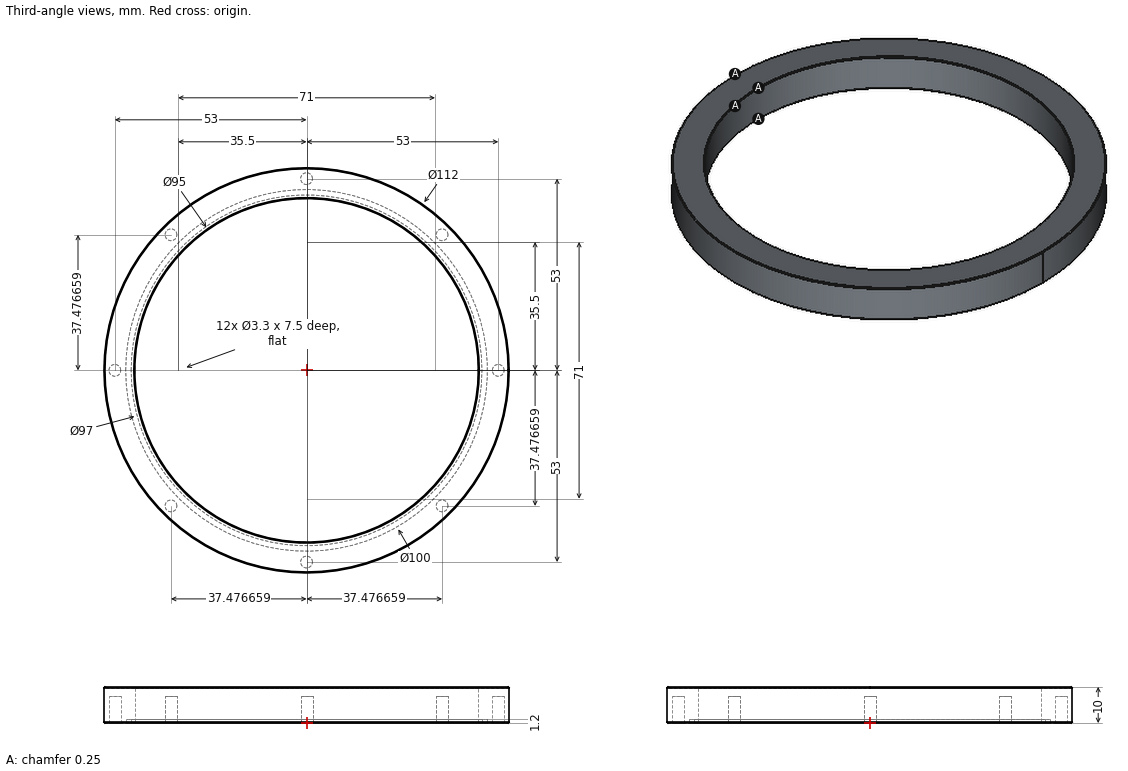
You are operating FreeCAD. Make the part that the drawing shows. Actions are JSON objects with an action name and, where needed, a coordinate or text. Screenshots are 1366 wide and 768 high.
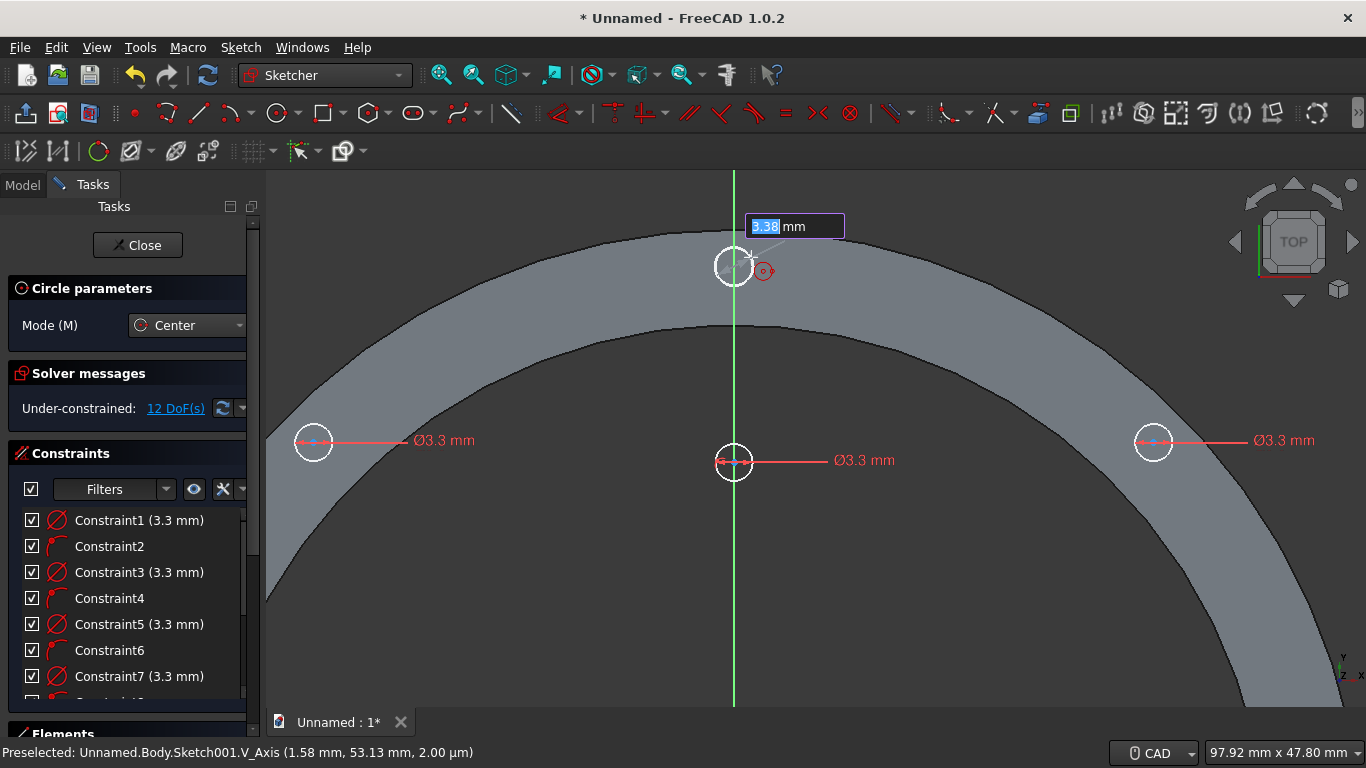
{"action": "type", "text": "3.3"}
{"action": "key", "text": "Return"}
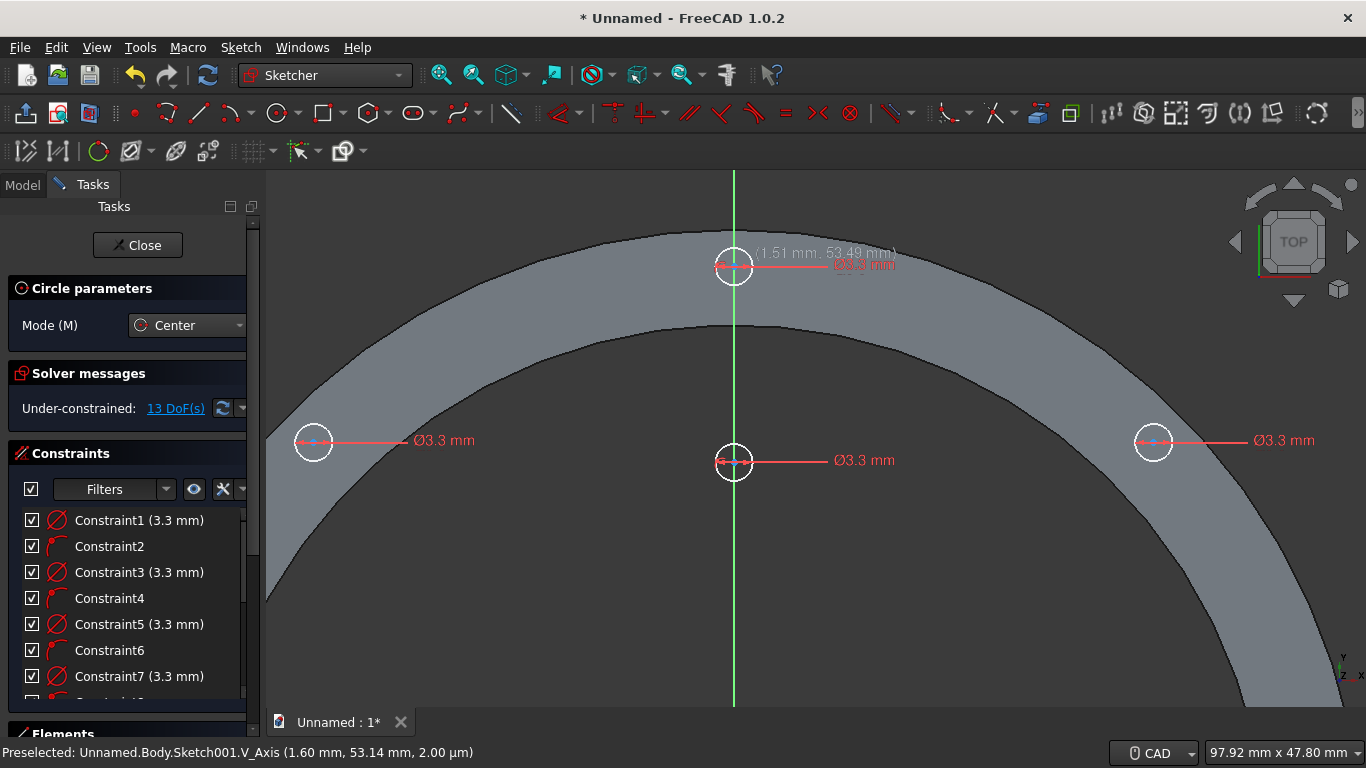
{"action": "scroll", "coordinate": [753, 257], "scroll_direction": "down", "scroll_amount": 6}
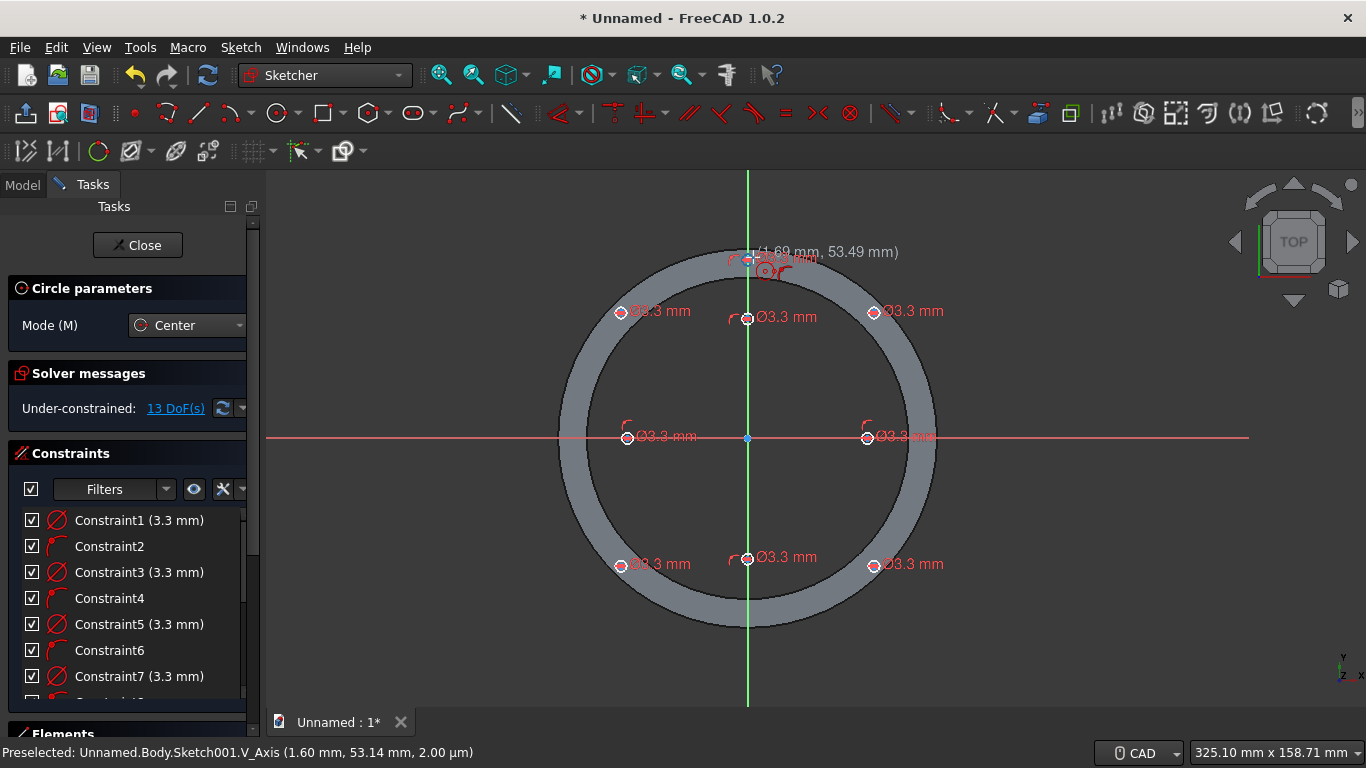
{"action": "scroll", "coordinate": [568, 438], "scroll_direction": "up", "scroll_amount": 8}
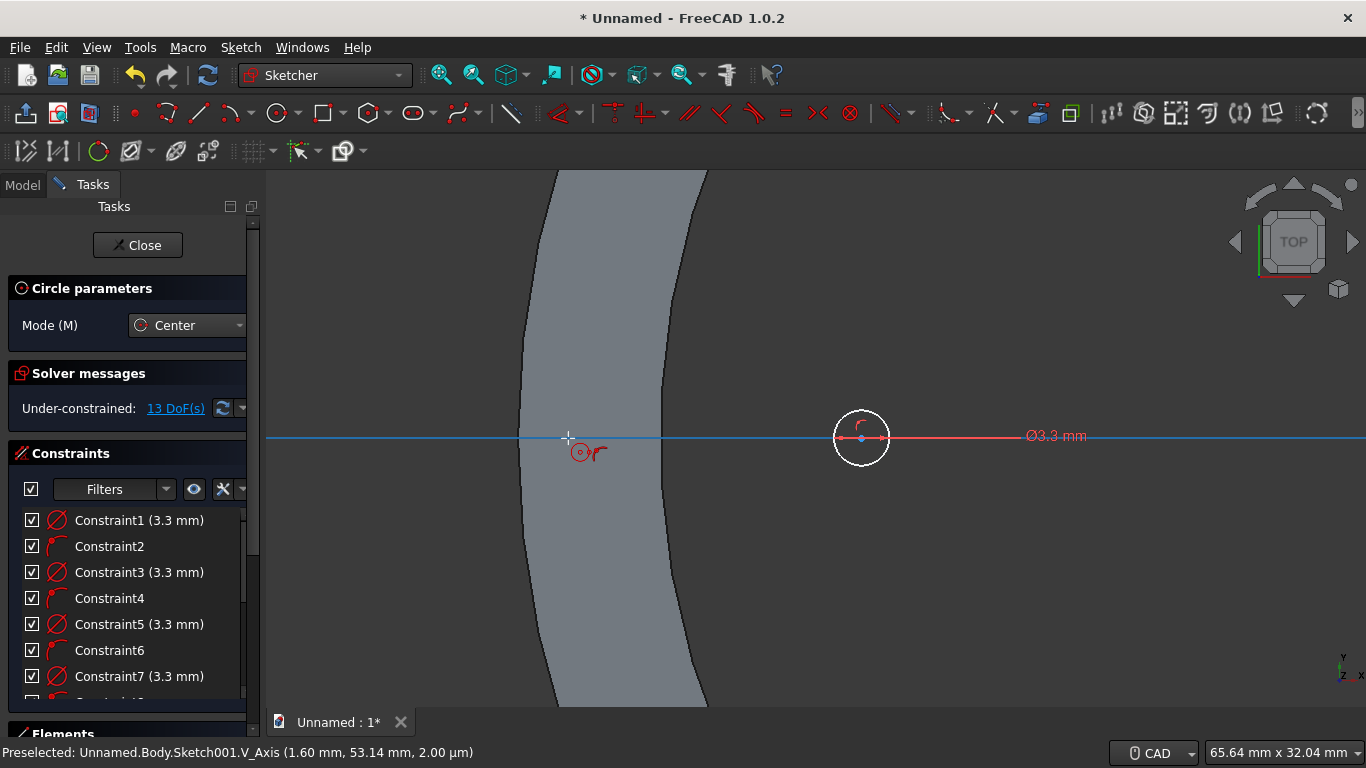
{"action": "scroll", "coordinate": [568, 439], "scroll_direction": "down", "scroll_amount": 8}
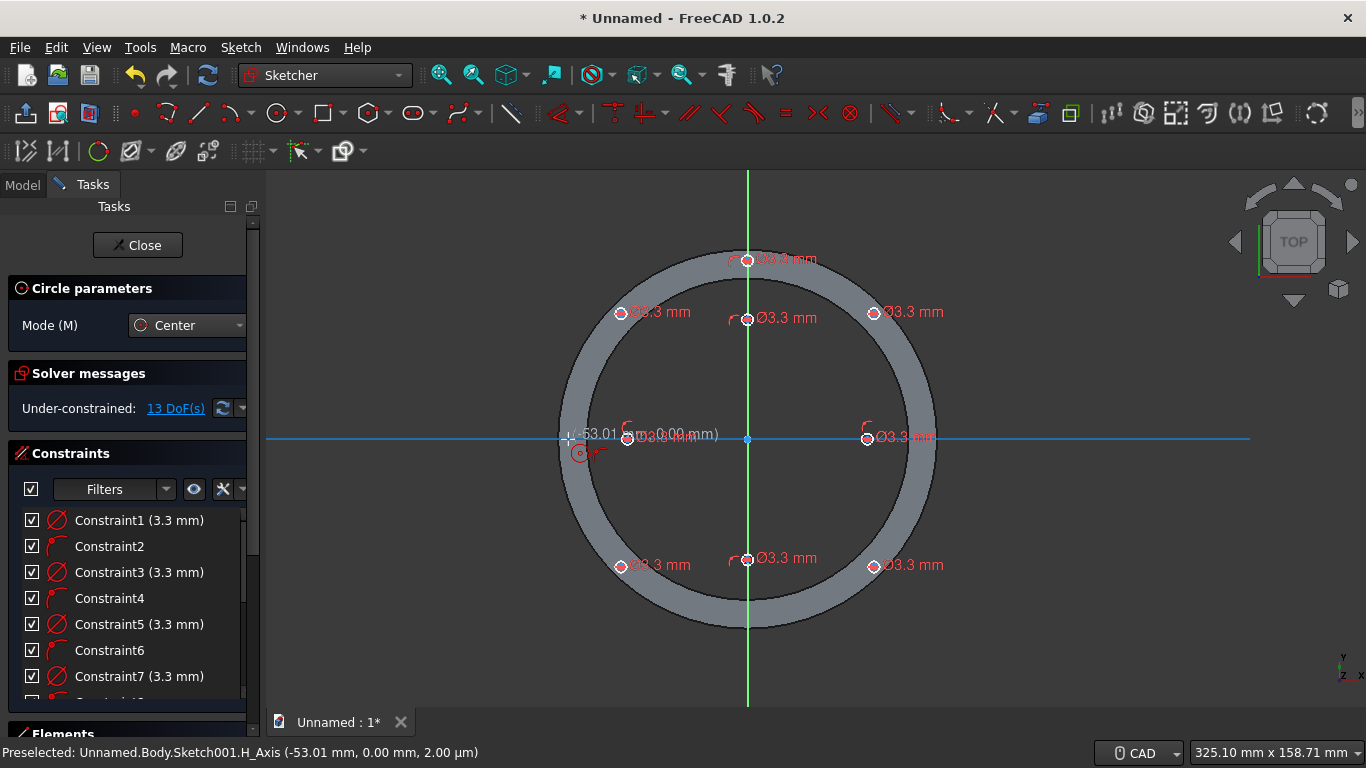
{"action": "left_click", "coordinate": [568, 439]}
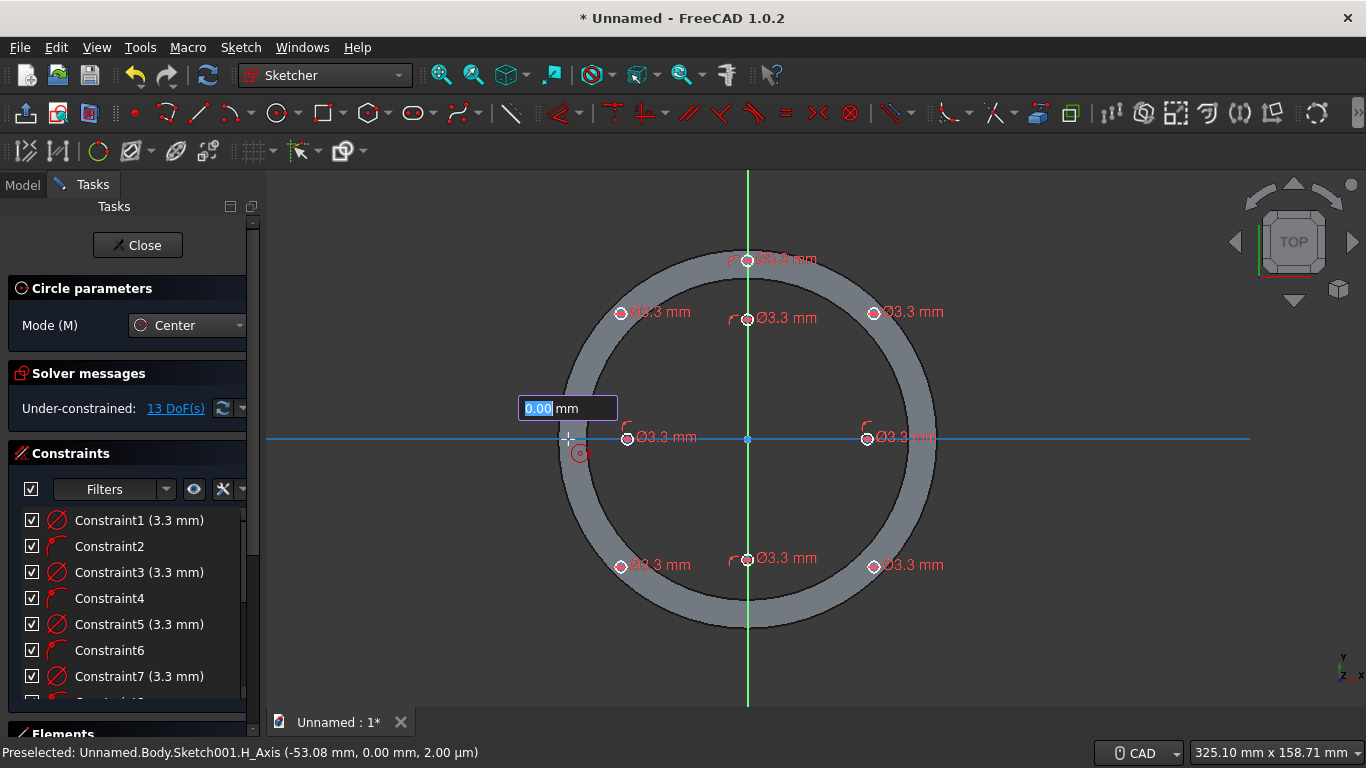
{"action": "scroll", "coordinate": [566, 444], "scroll_direction": "up", "scroll_amount": 6}
{"action": "mouse_move", "coordinate": [567, 444]}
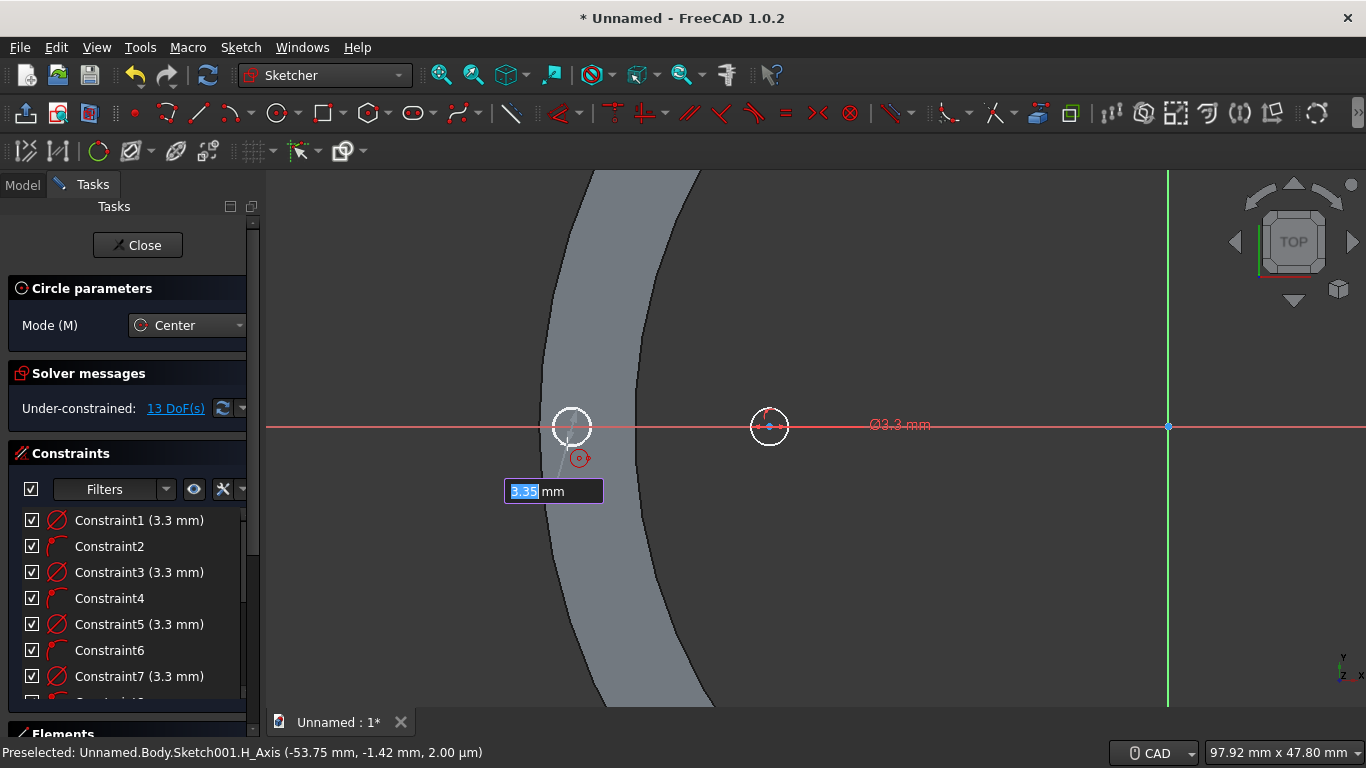
{"action": "type", "text": "3.3"}
{"action": "key", "text": "Return"}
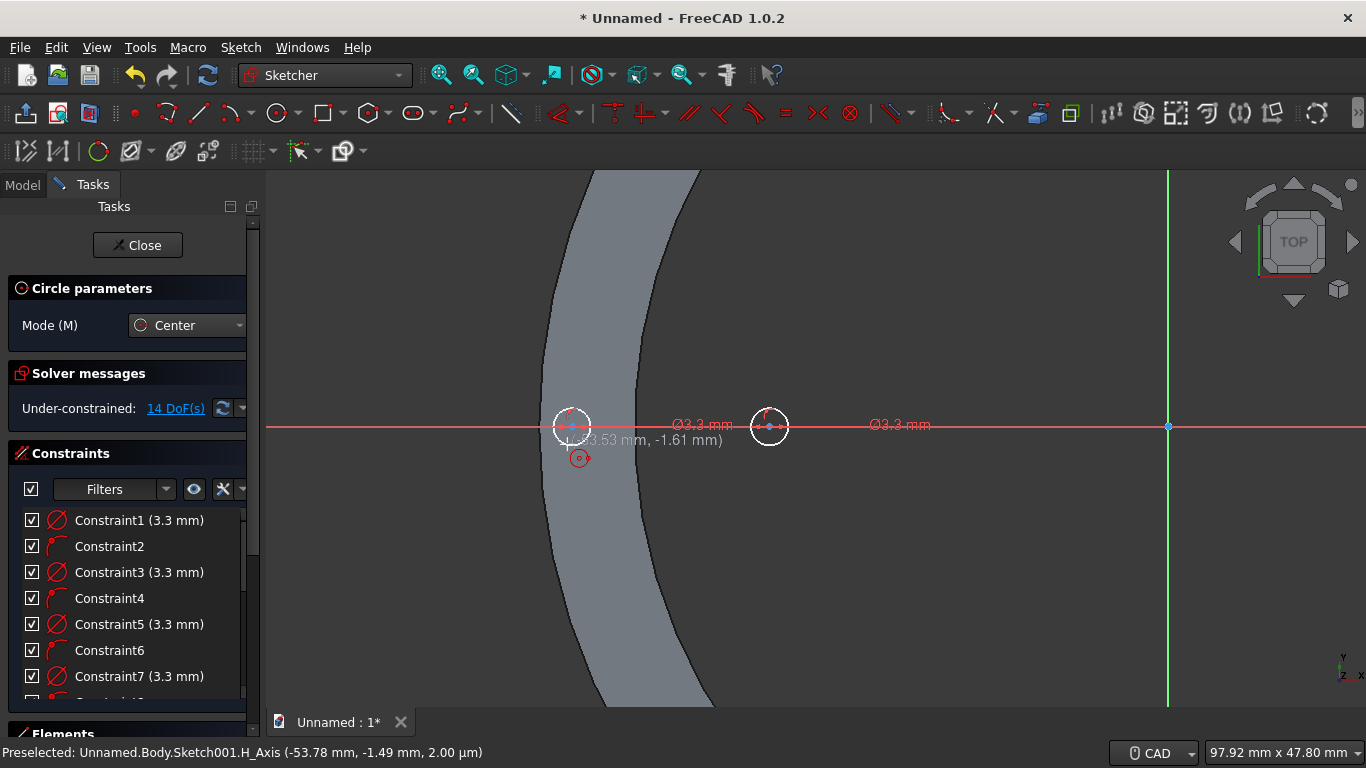
{"action": "scroll", "coordinate": [566, 444], "scroll_direction": "down", "scroll_amount": 6}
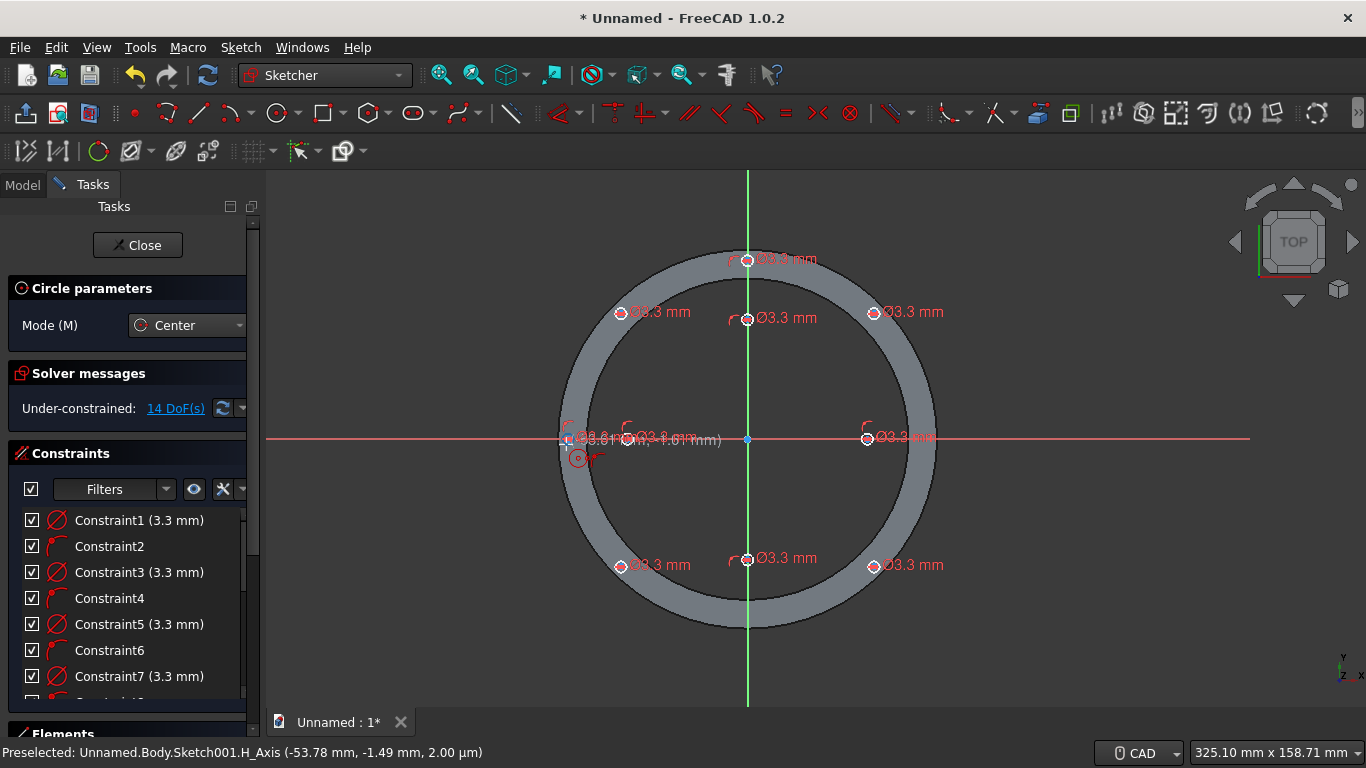
{"action": "scroll", "coordinate": [748, 619], "scroll_direction": "up", "scroll_amount": 8}